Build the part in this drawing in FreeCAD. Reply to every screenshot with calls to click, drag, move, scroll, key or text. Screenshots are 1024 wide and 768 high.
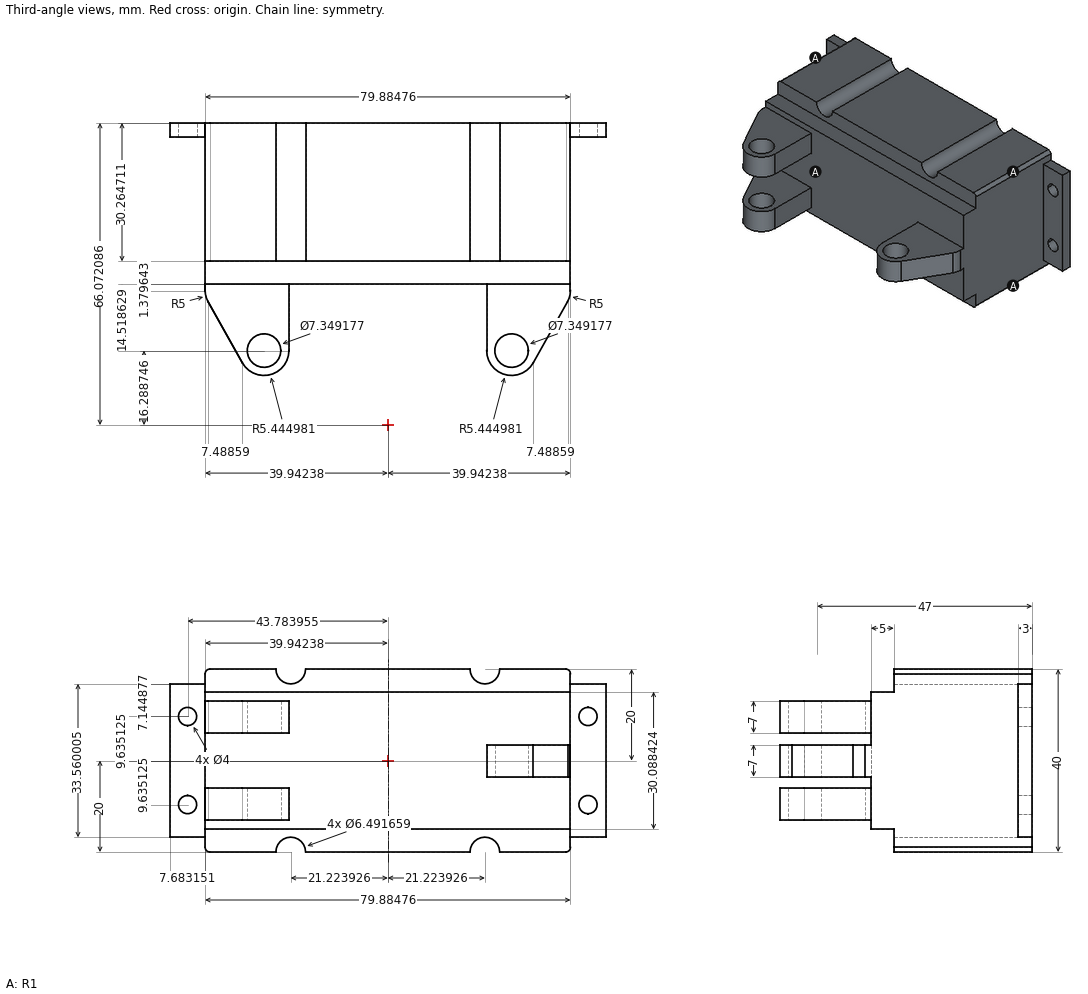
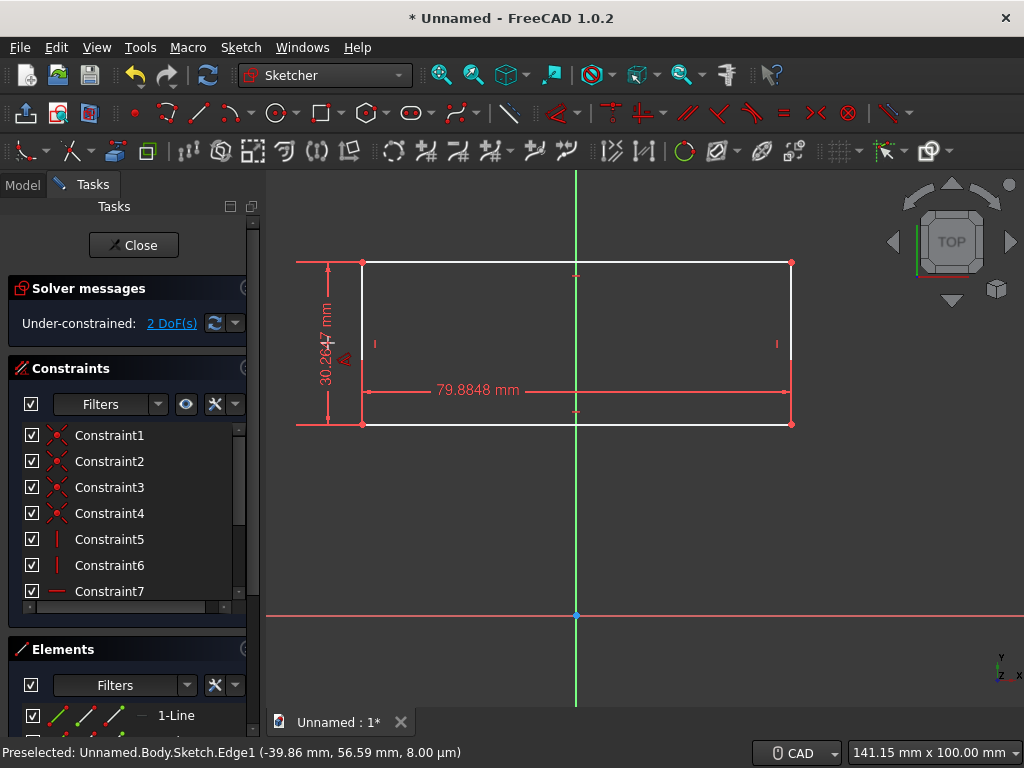
click(362, 262)
click(469, 650)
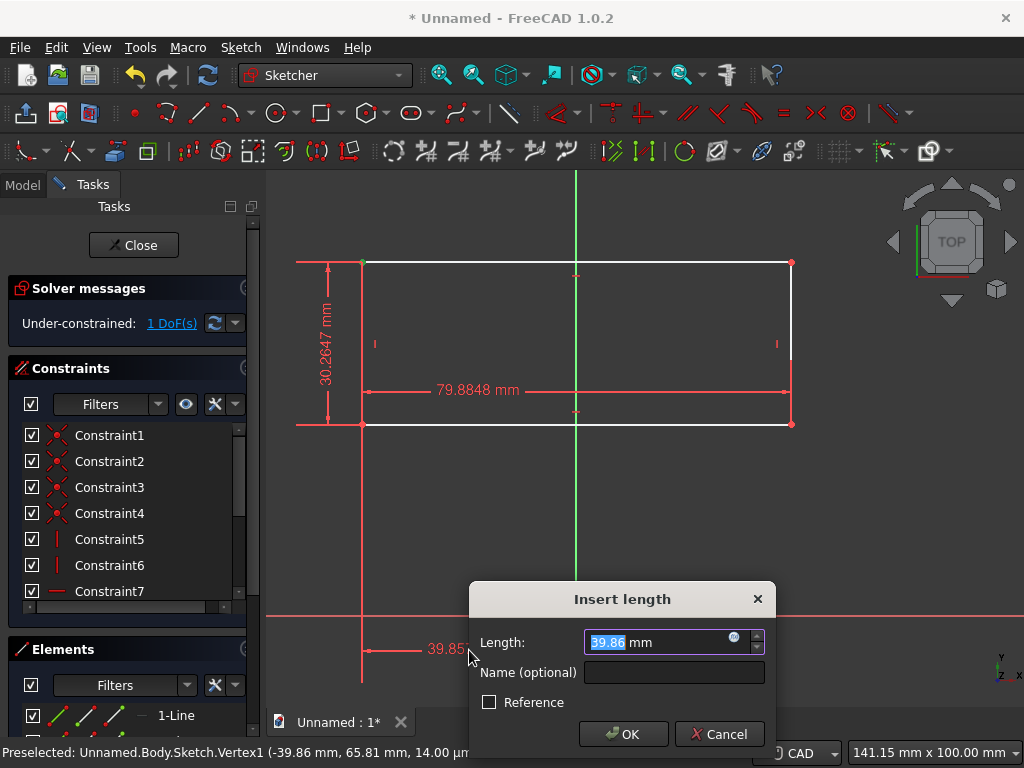
text(39.94238)
key(Return)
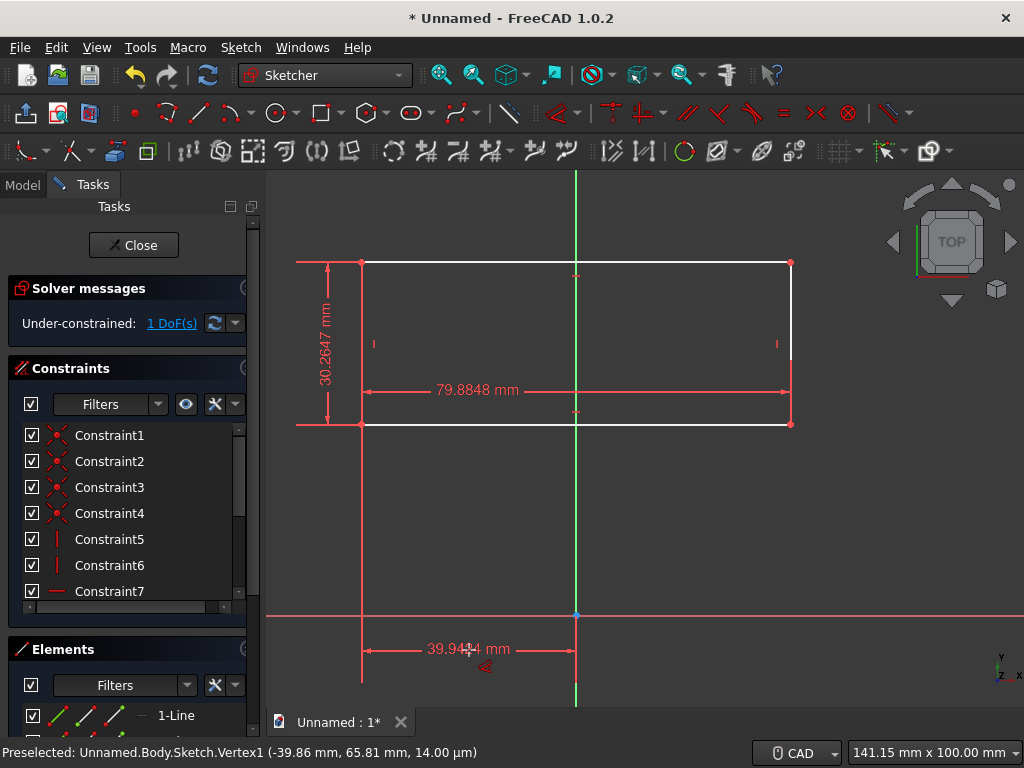
click(362, 262)
click(328, 439)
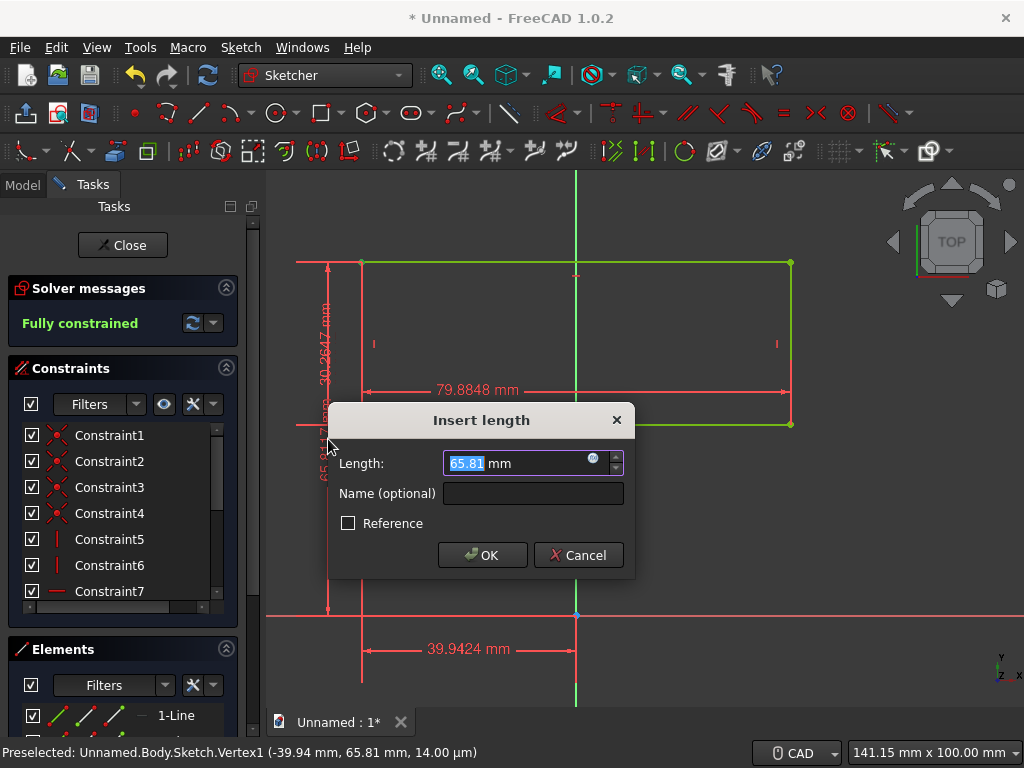
text(66.072086)
key(Return)
key(Escape)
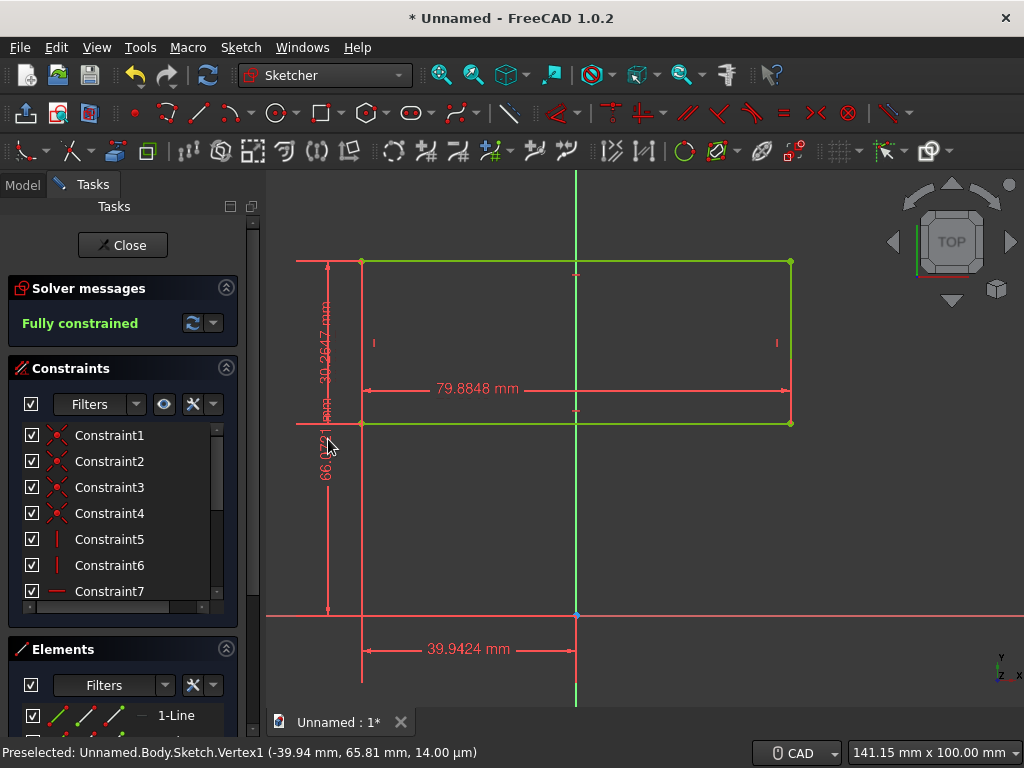
click(123, 245)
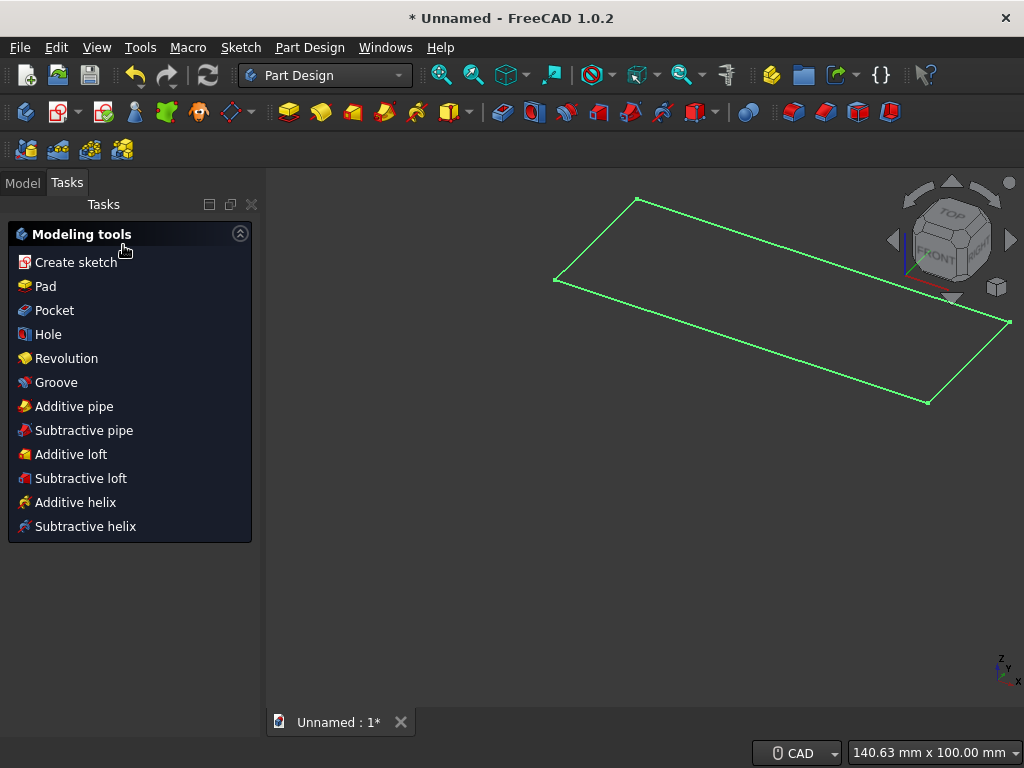
click(290, 112)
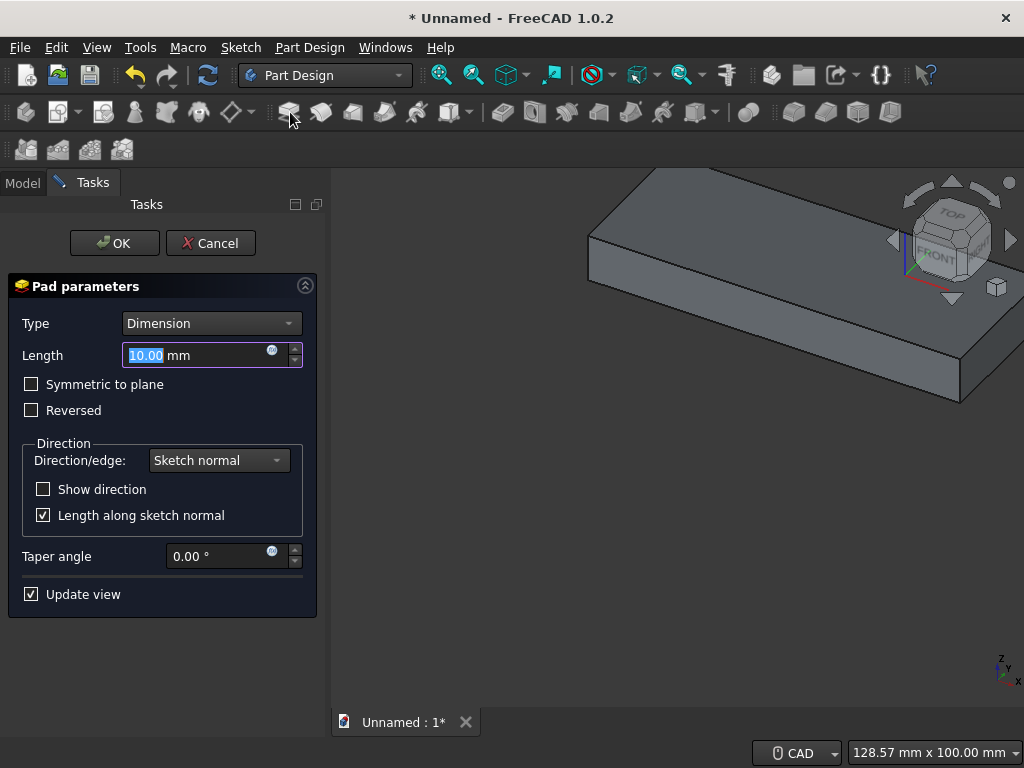
text(40)
key(Tab)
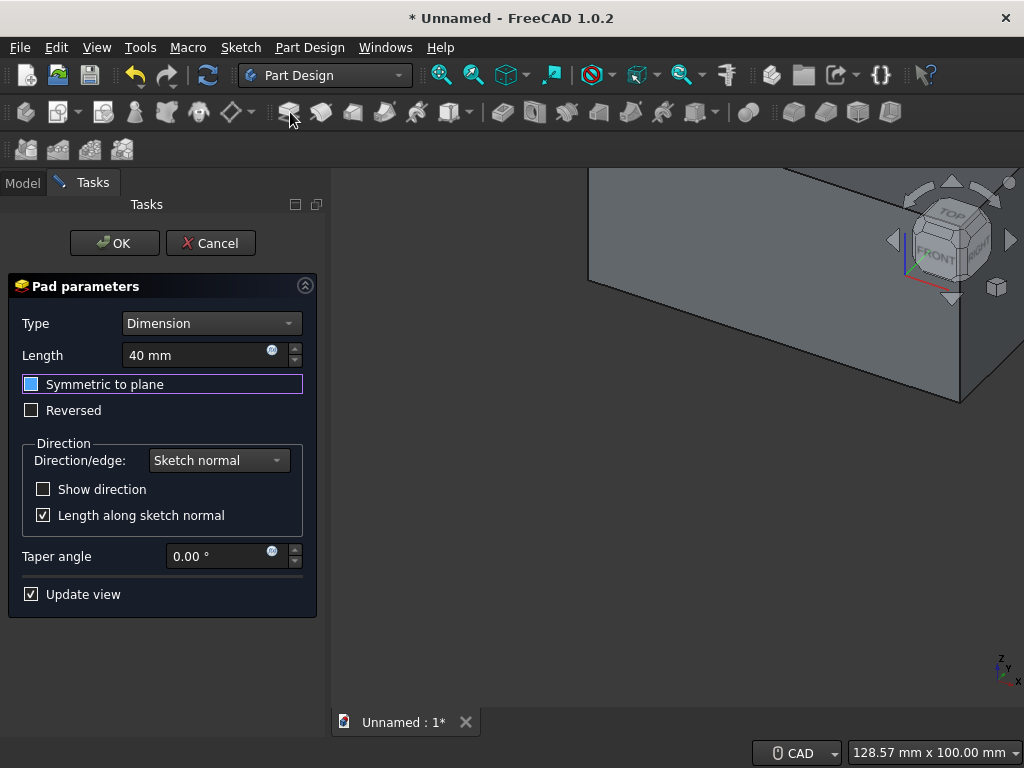
click(30, 384)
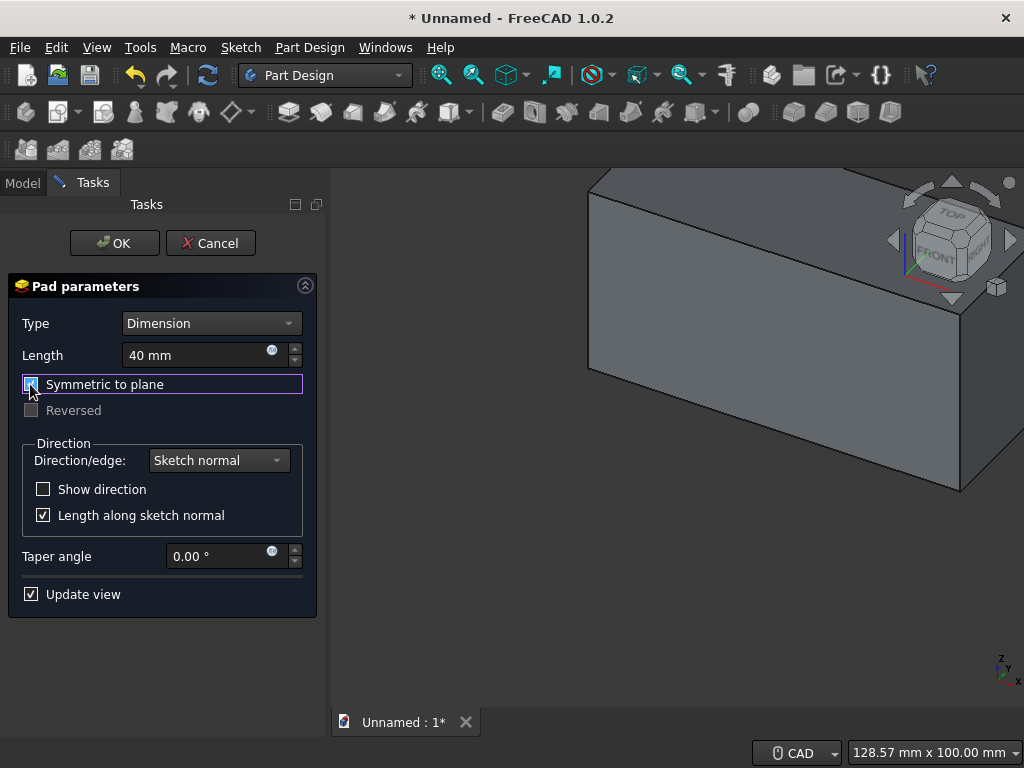
click(115, 243)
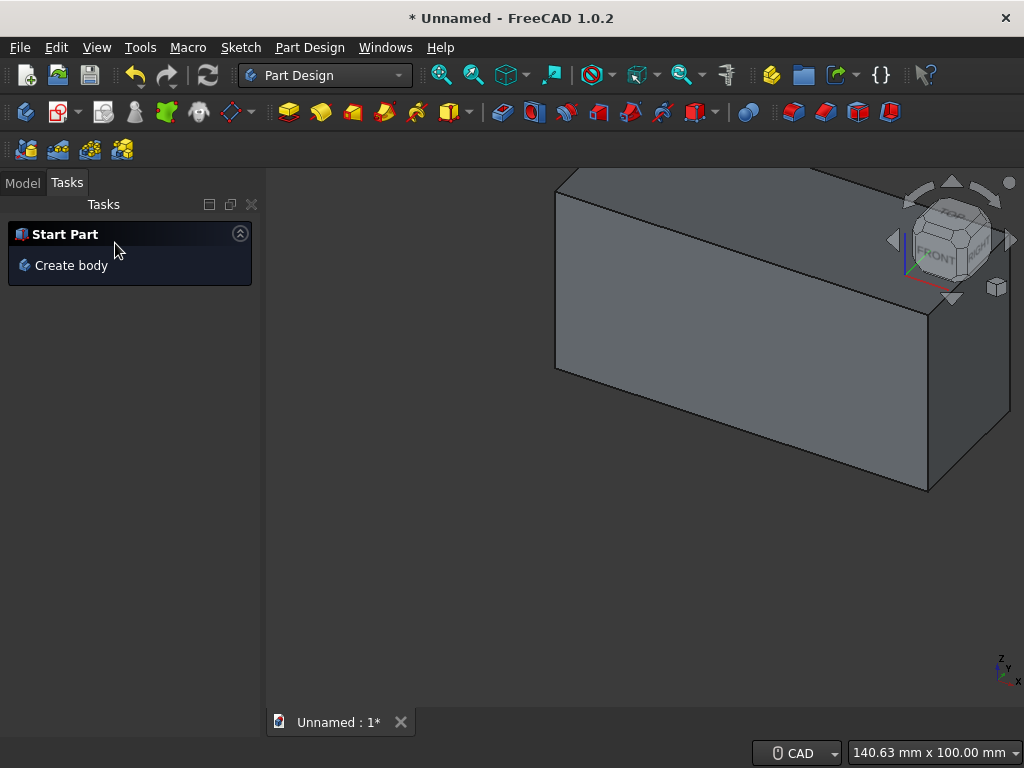
click(442, 76)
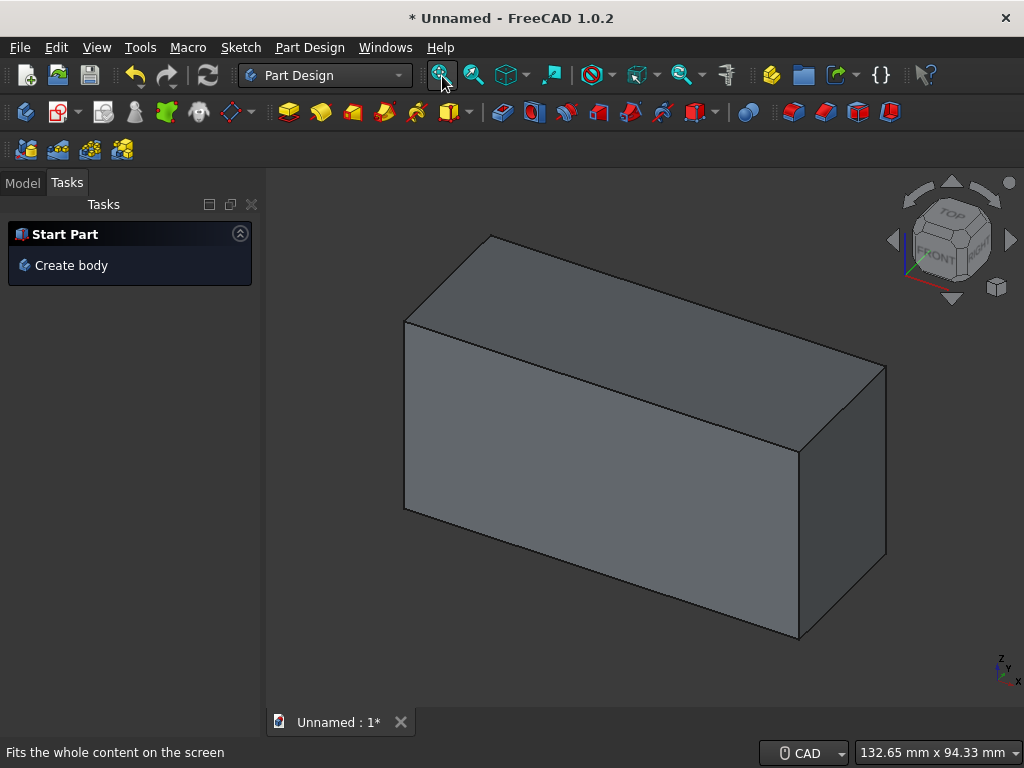
click(658, 498)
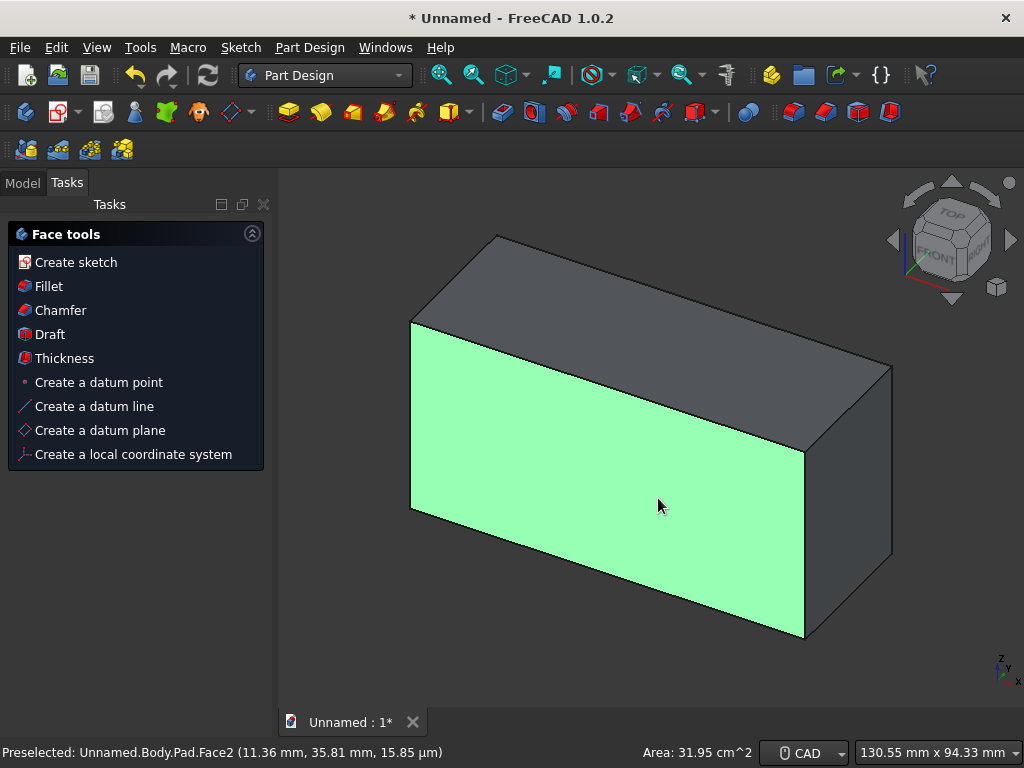
click(58, 112)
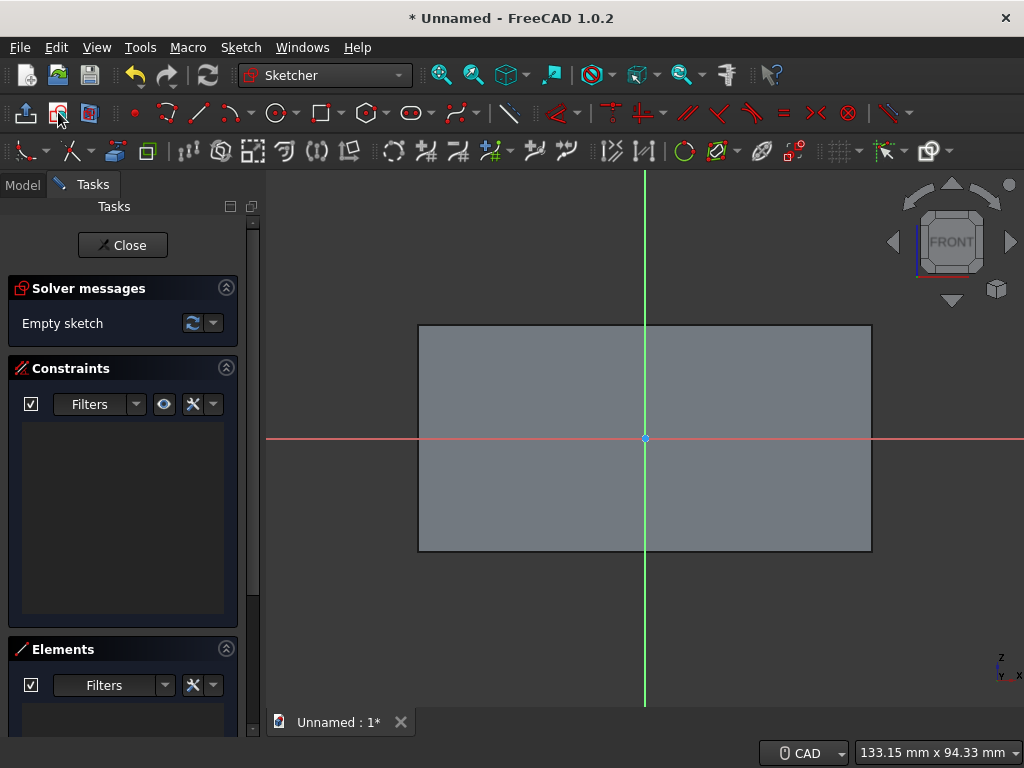
scroll(294, 438, down, 1)